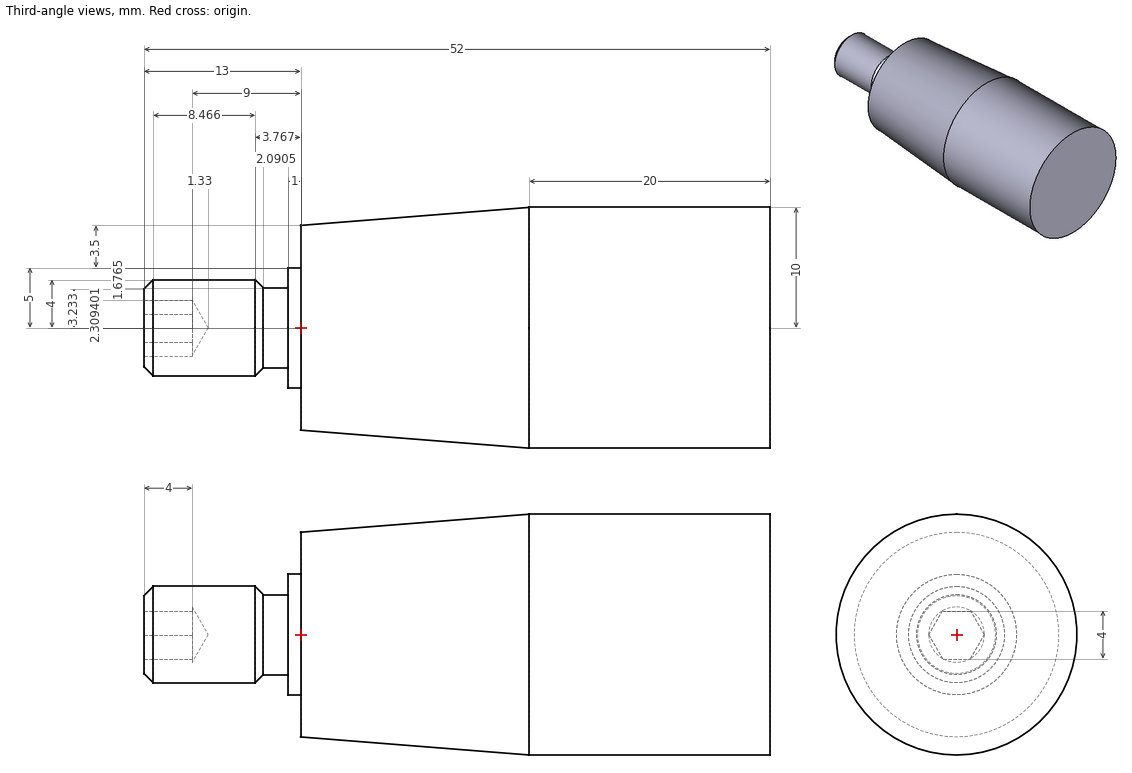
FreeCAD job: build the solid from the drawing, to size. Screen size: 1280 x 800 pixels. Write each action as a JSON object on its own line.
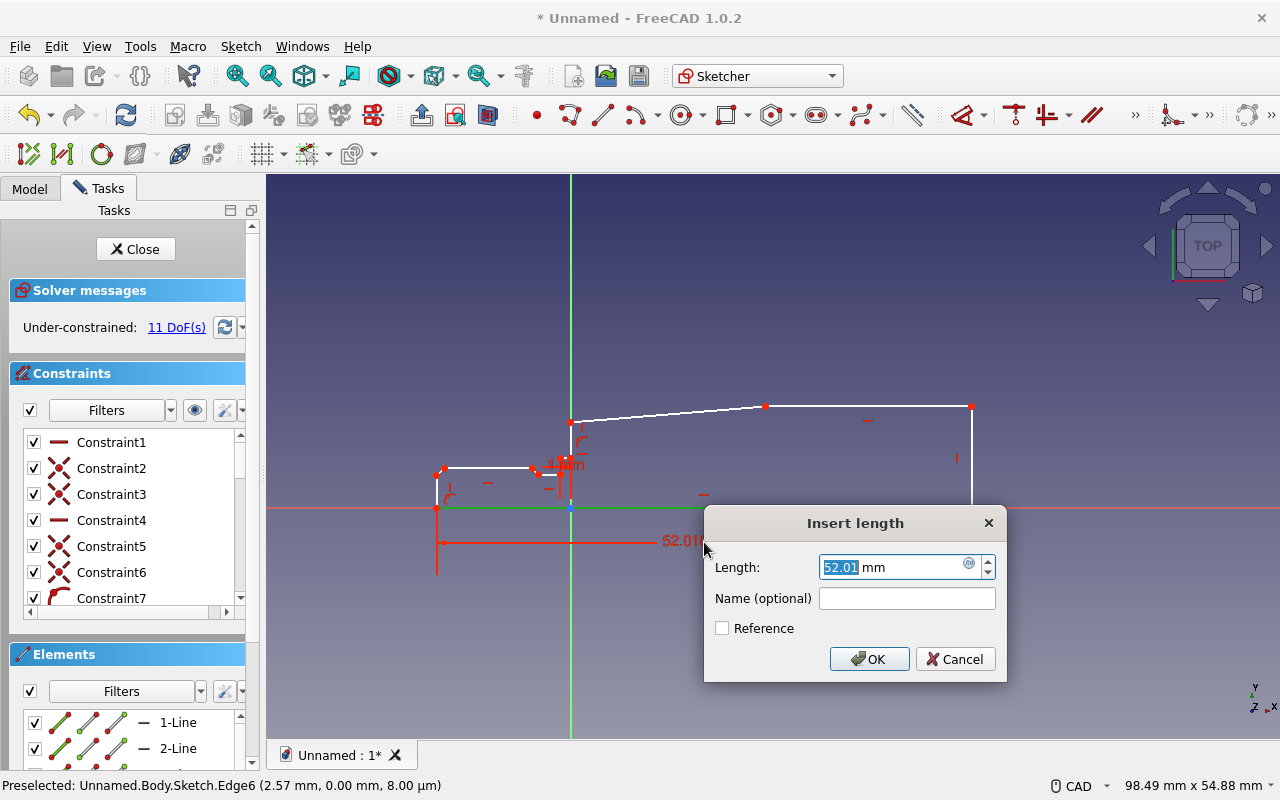
{"action": "type", "text": "52"}
{"action": "key", "text": "Return"}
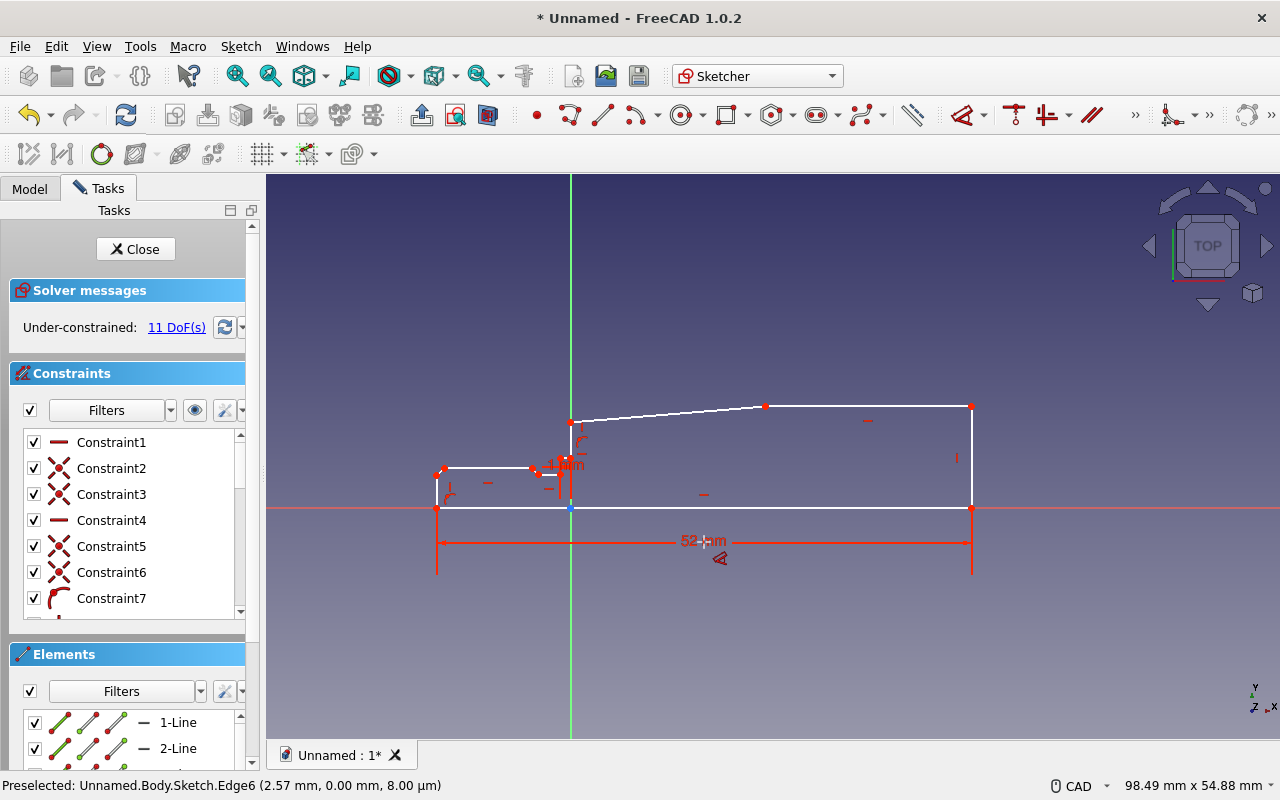
{"action": "left_click", "coordinate": [972, 478]}
{"action": "left_click", "coordinate": [1006, 457]}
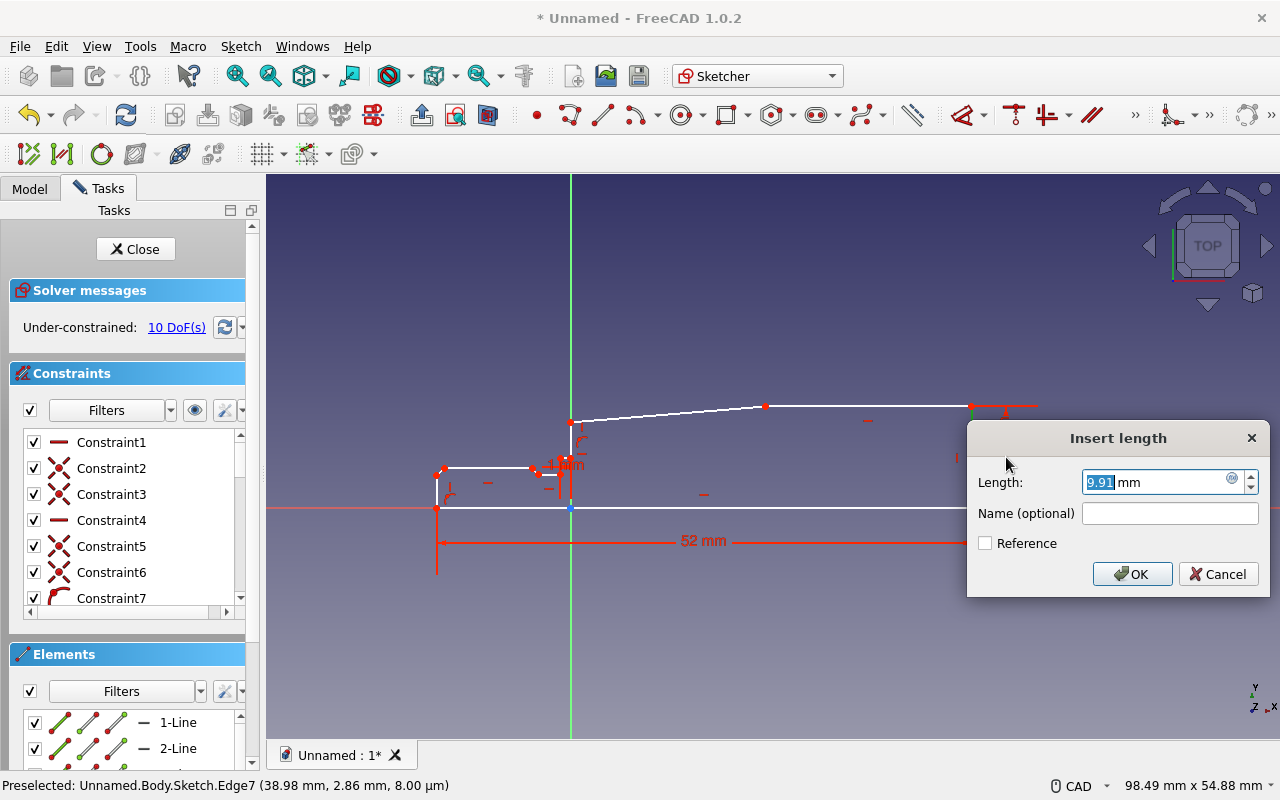
{"action": "type", "text": "10"}
{"action": "key", "text": "Return"}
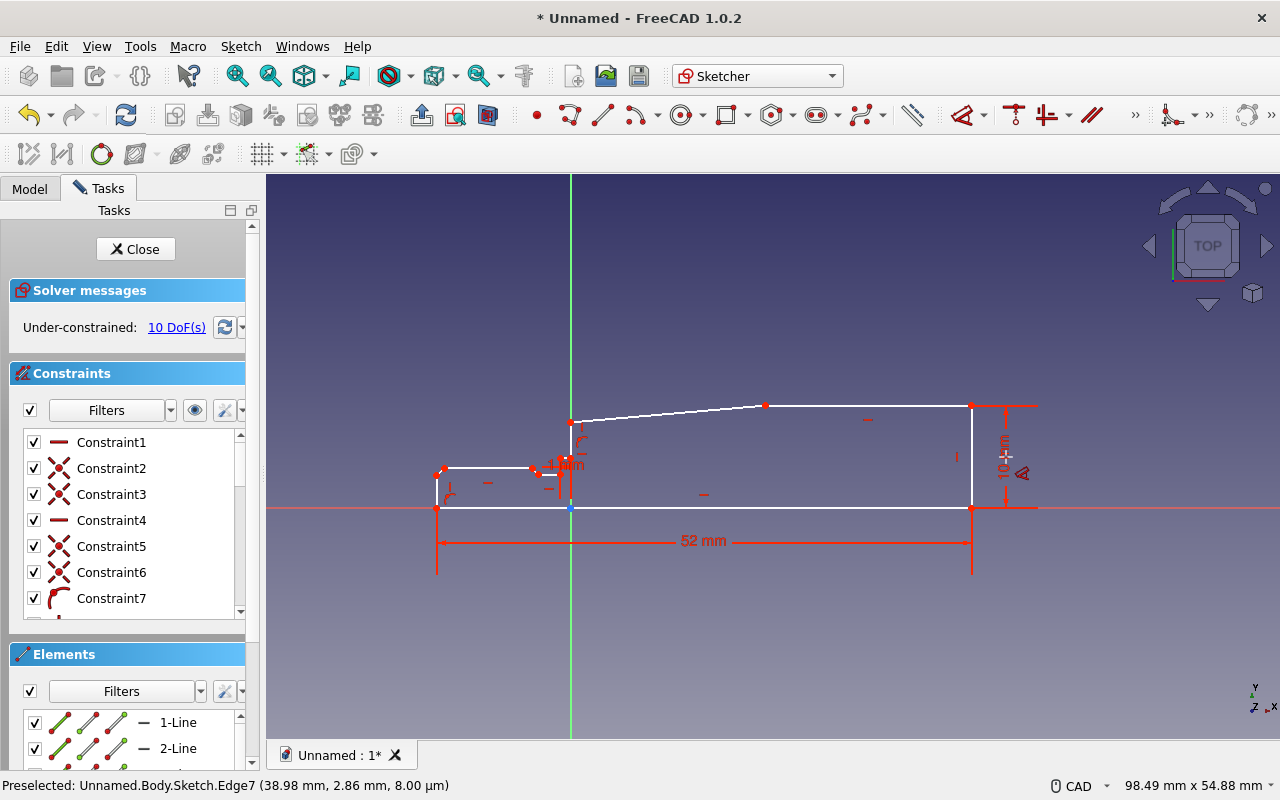
{"action": "left_click", "coordinate": [910, 406]}
{"action": "left_click", "coordinate": [869, 372]}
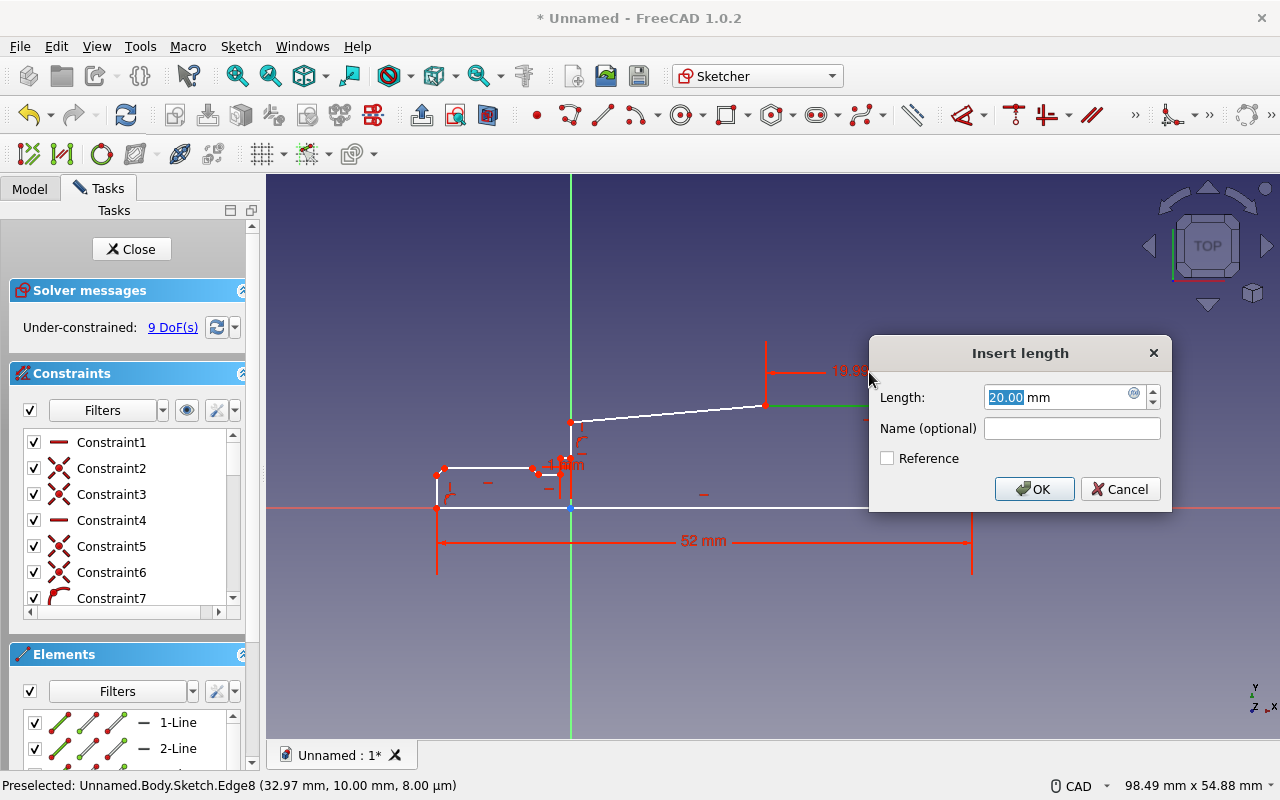
{"action": "type", "text": "20"}
{"action": "key", "text": "Return"}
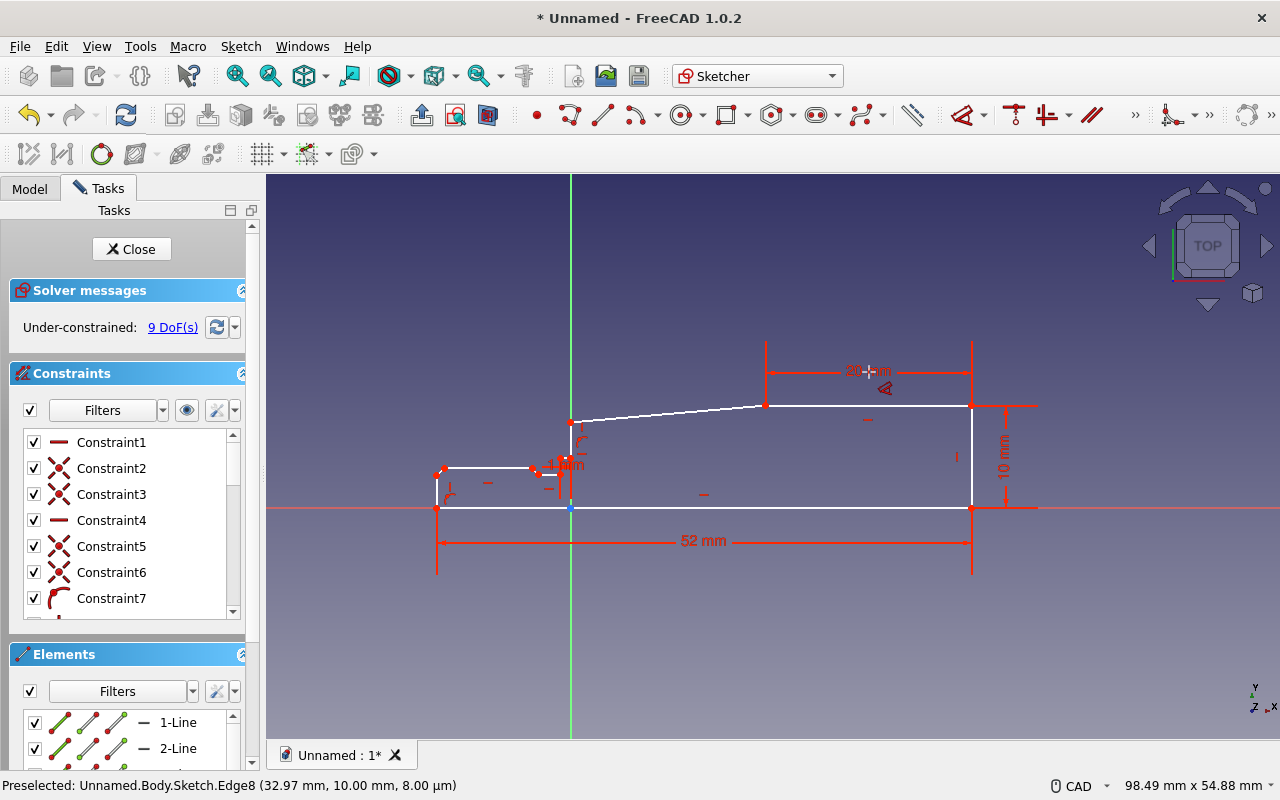
{"action": "scroll", "coordinate": [532, 468], "scroll_direction": "up", "scroll_amount": 2}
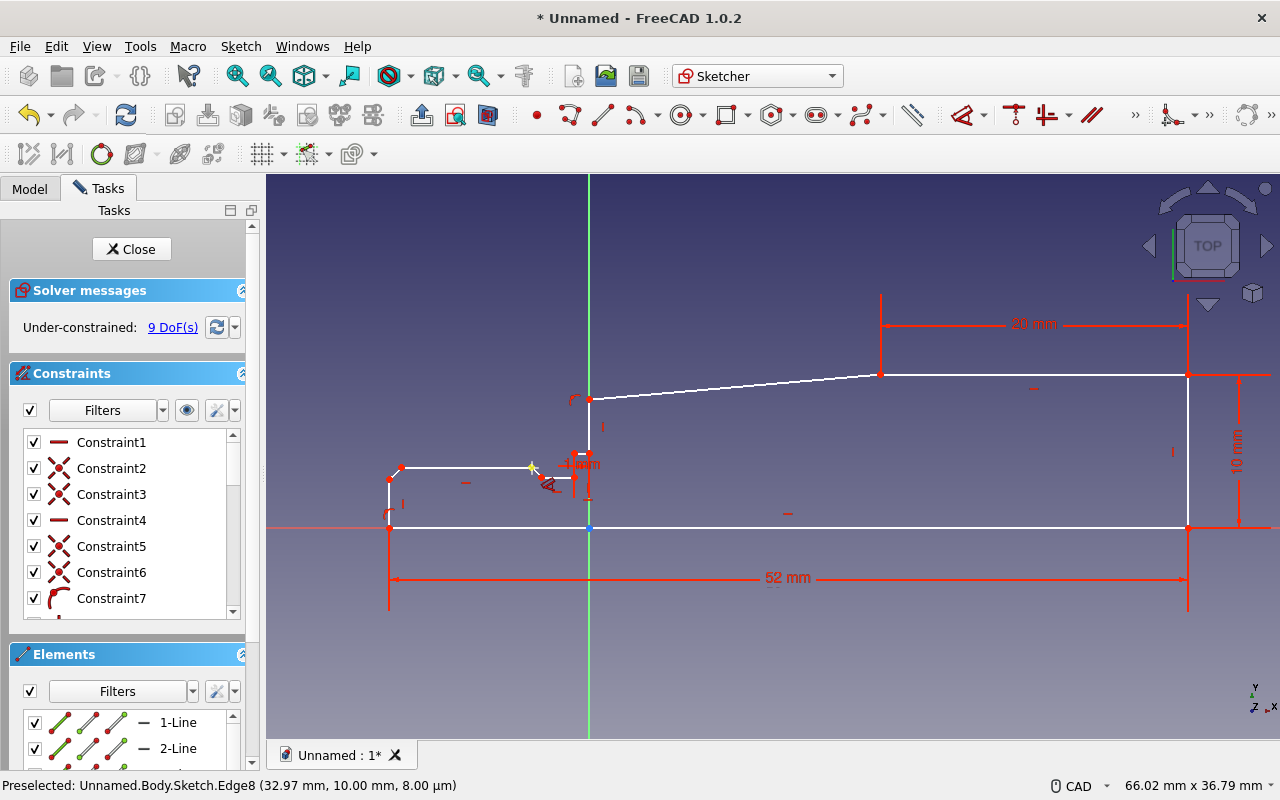
{"action": "left_click", "coordinate": [532, 468]}
{"action": "left_click", "coordinate": [498, 498]}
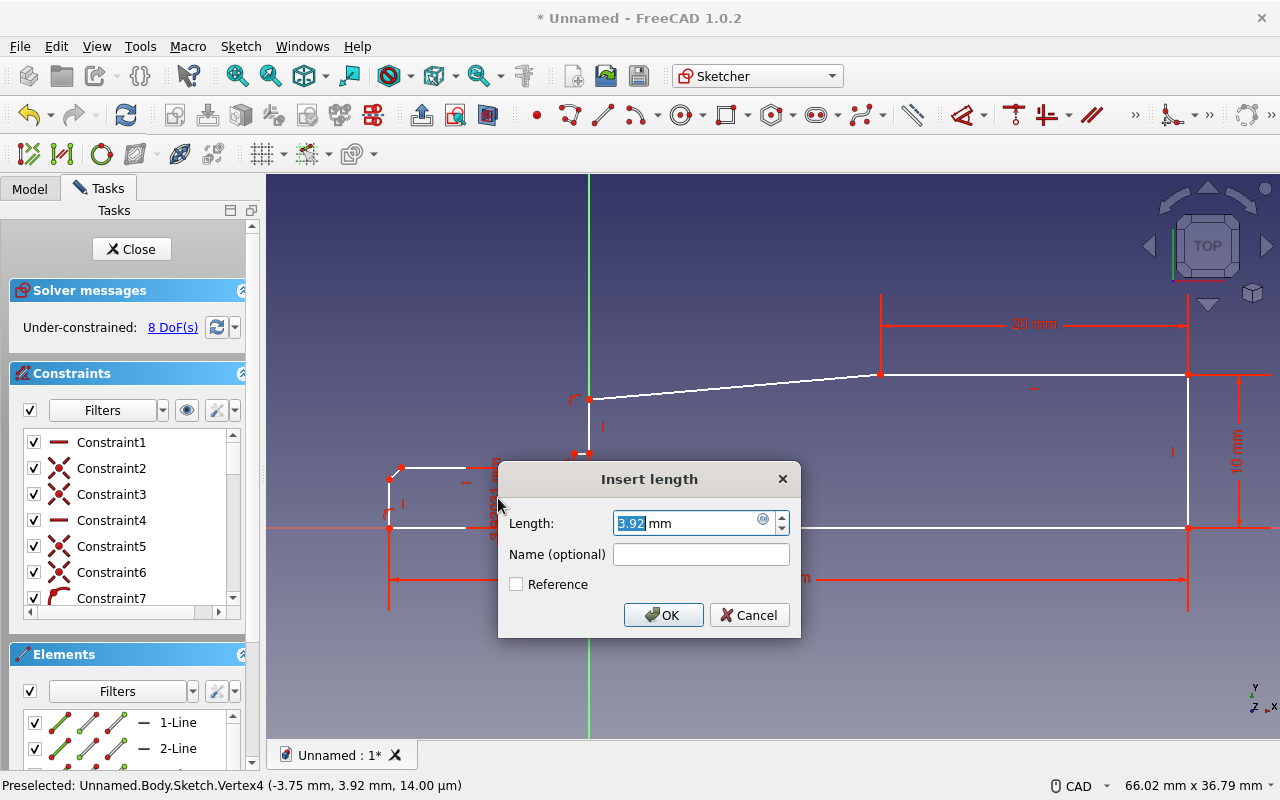
{"action": "type", "text": "4"}
{"action": "key", "text": "Return"}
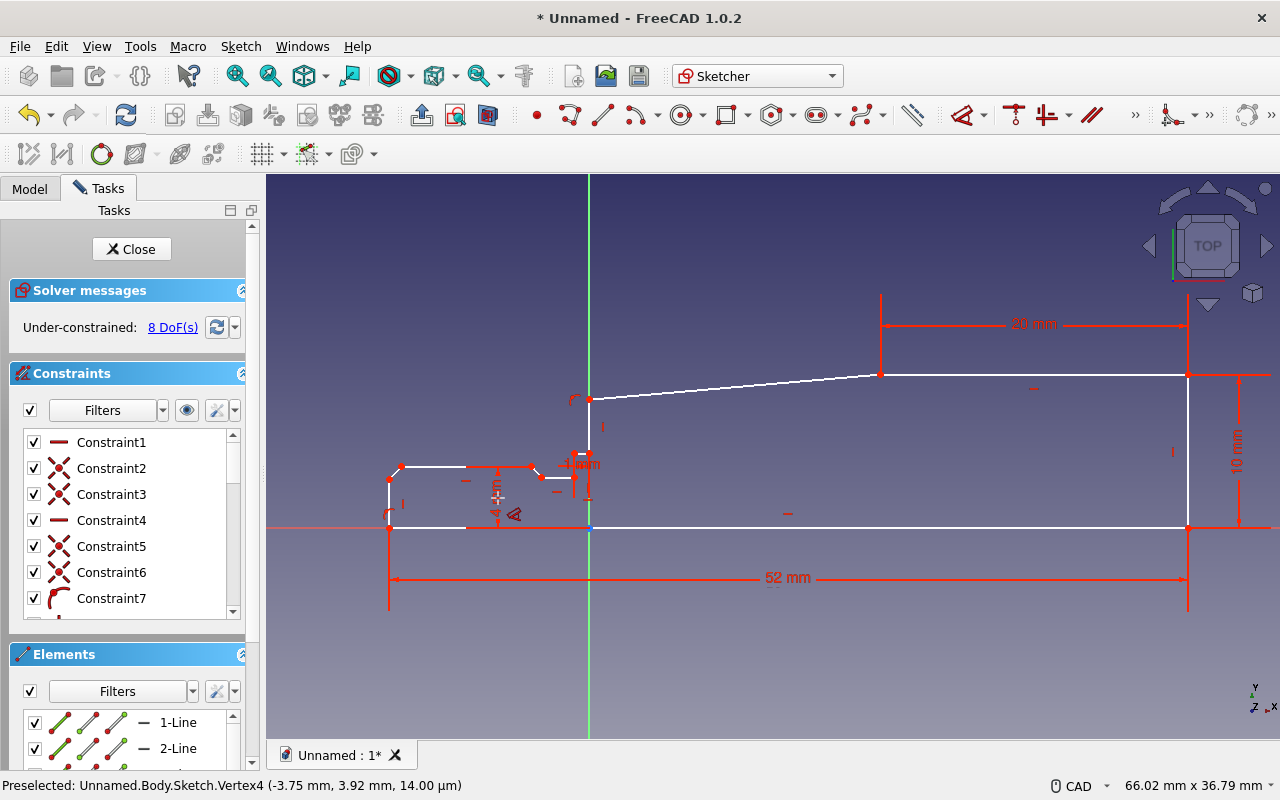
{"action": "left_click", "coordinate": [589, 453]}
{"action": "left_click", "coordinate": [623, 491]}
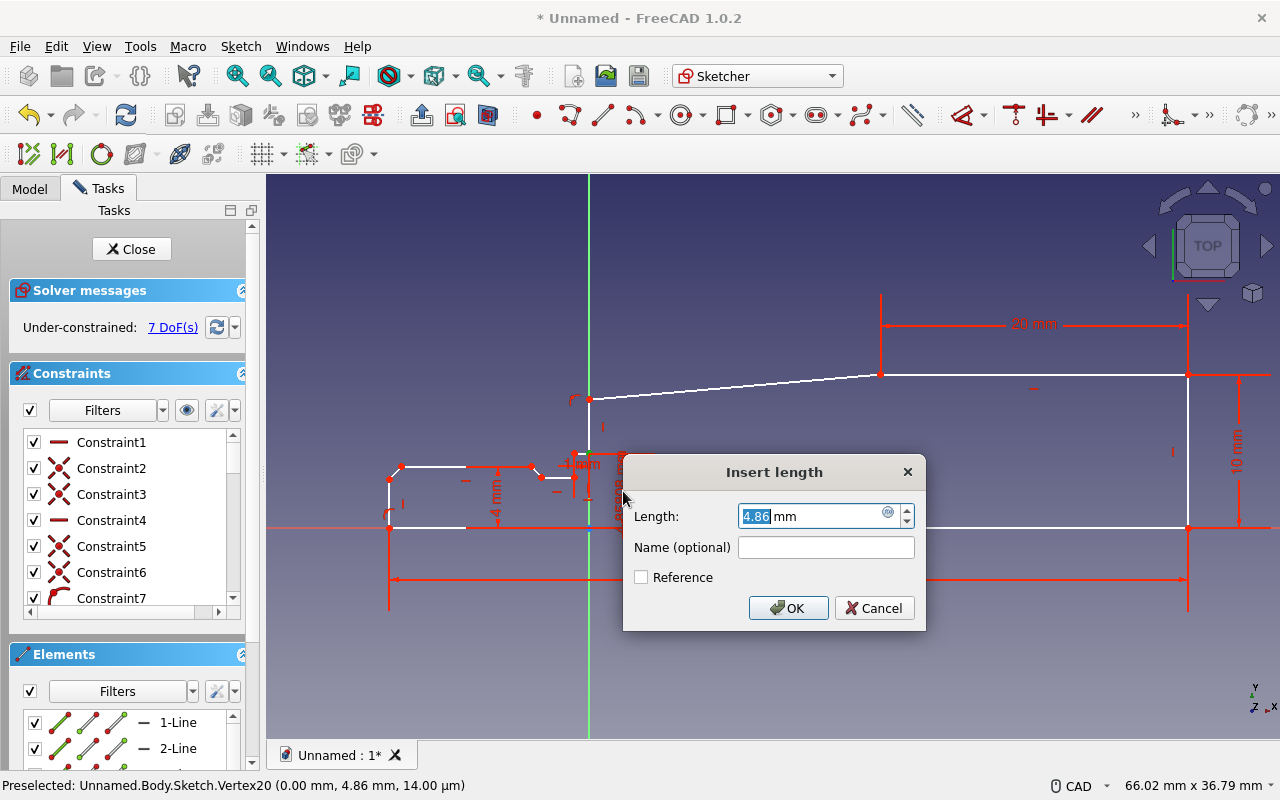
{"action": "type", "text": "5"}
{"action": "key", "text": "Return"}